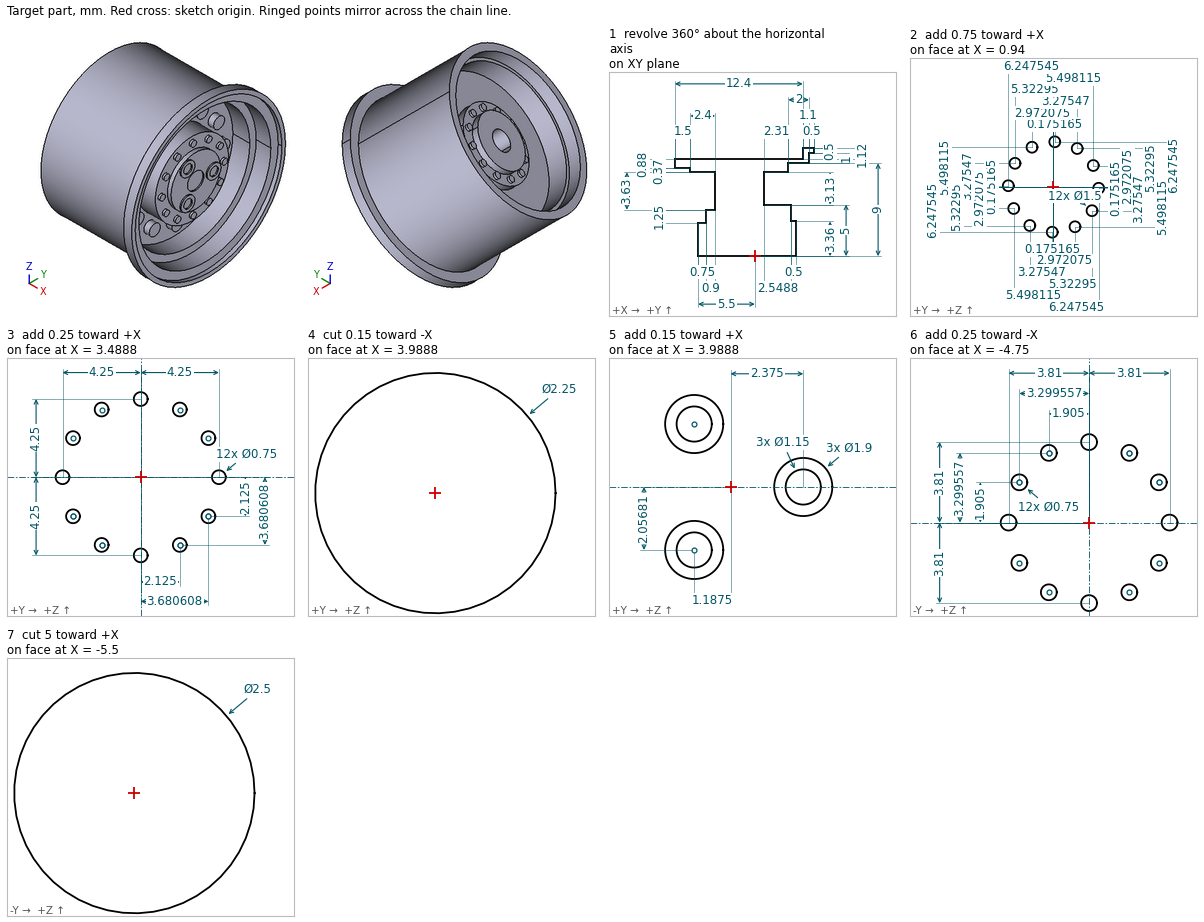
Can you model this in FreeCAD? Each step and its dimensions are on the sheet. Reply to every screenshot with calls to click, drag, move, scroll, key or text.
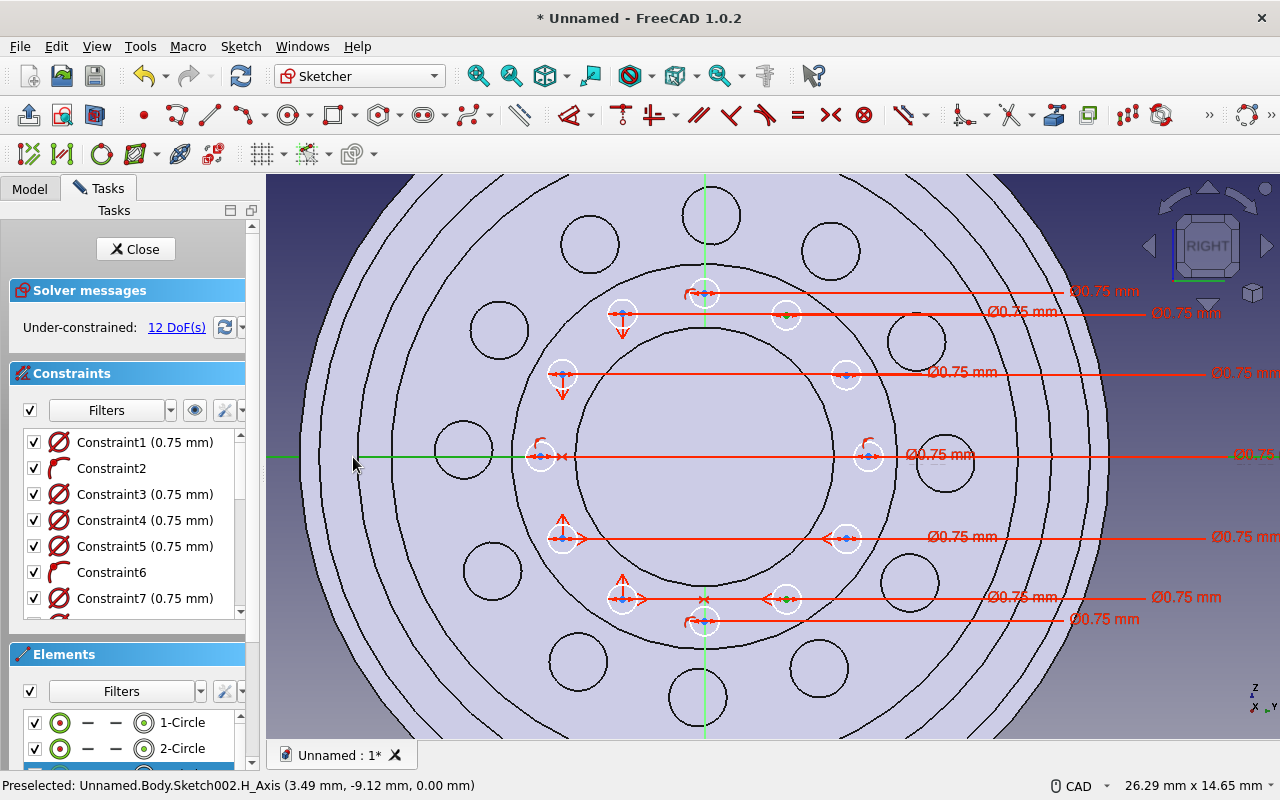
click(831, 116)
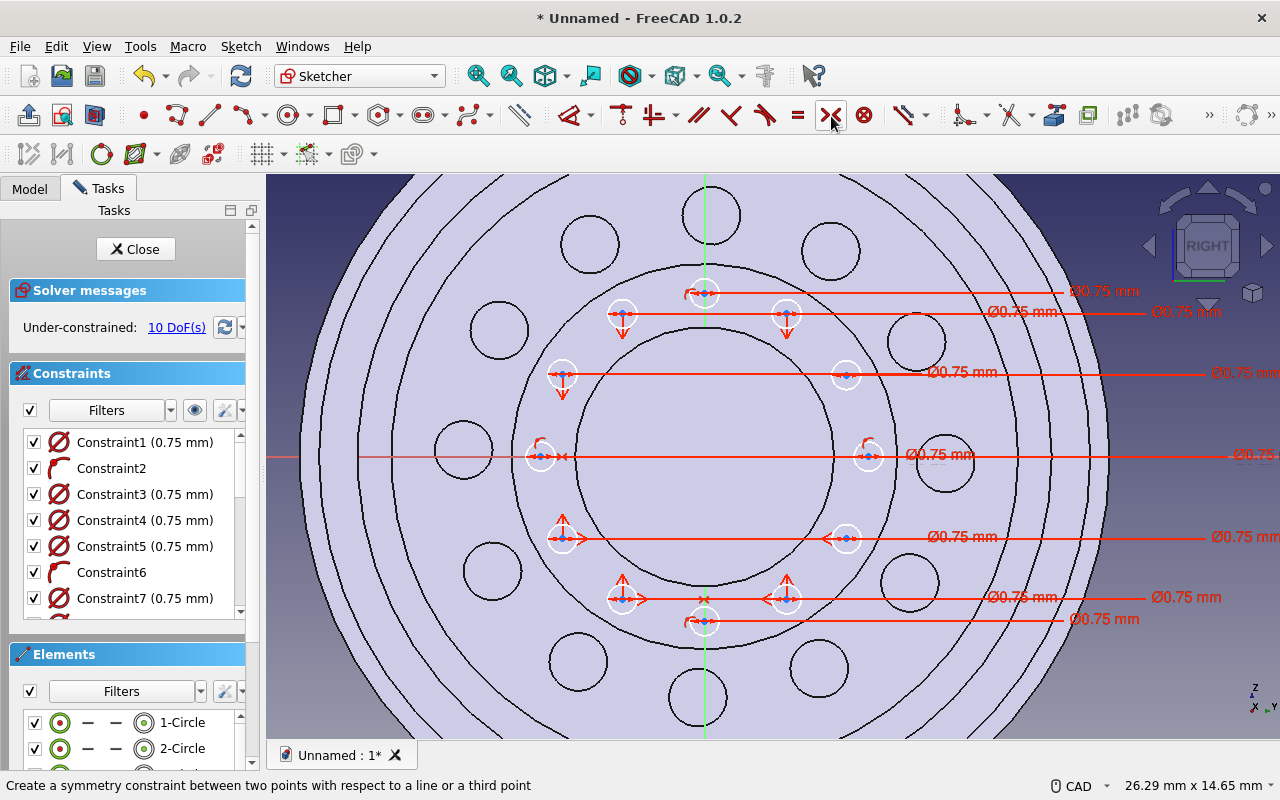
click(847, 539)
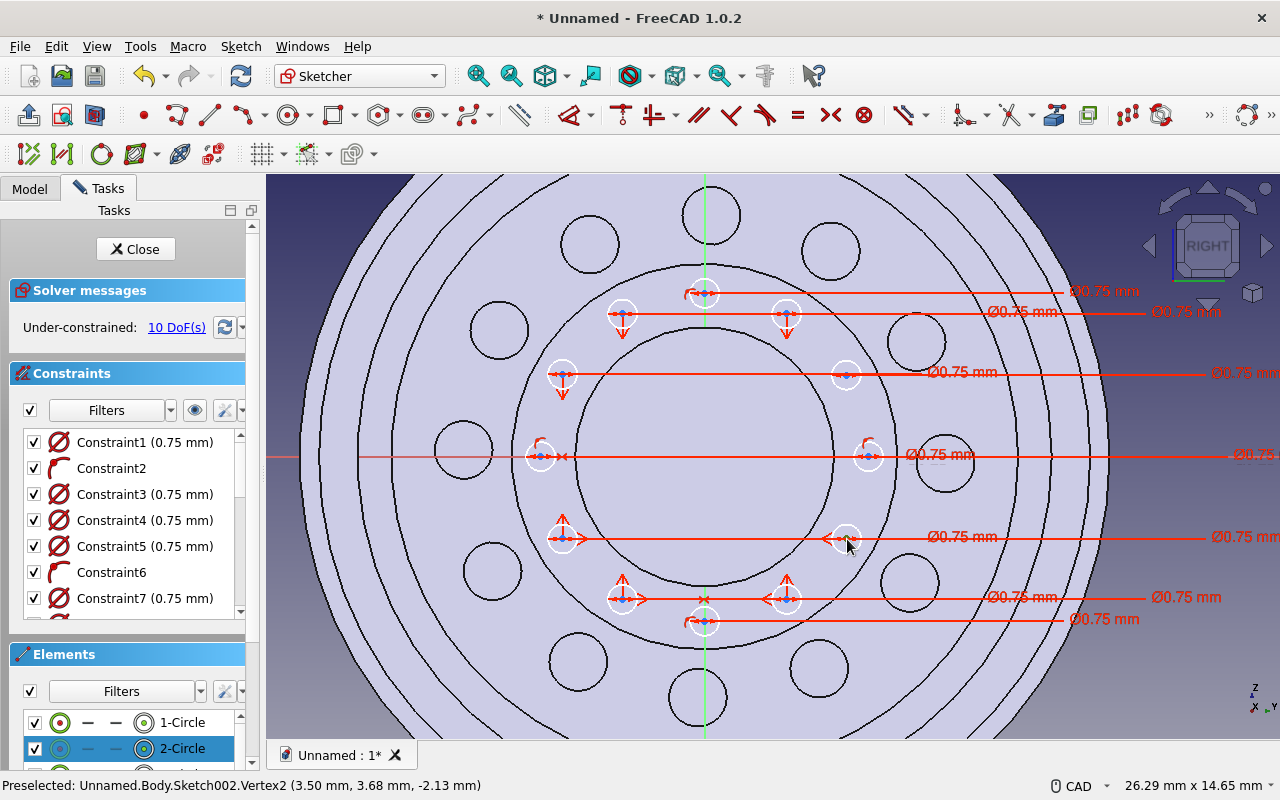
click(846, 375)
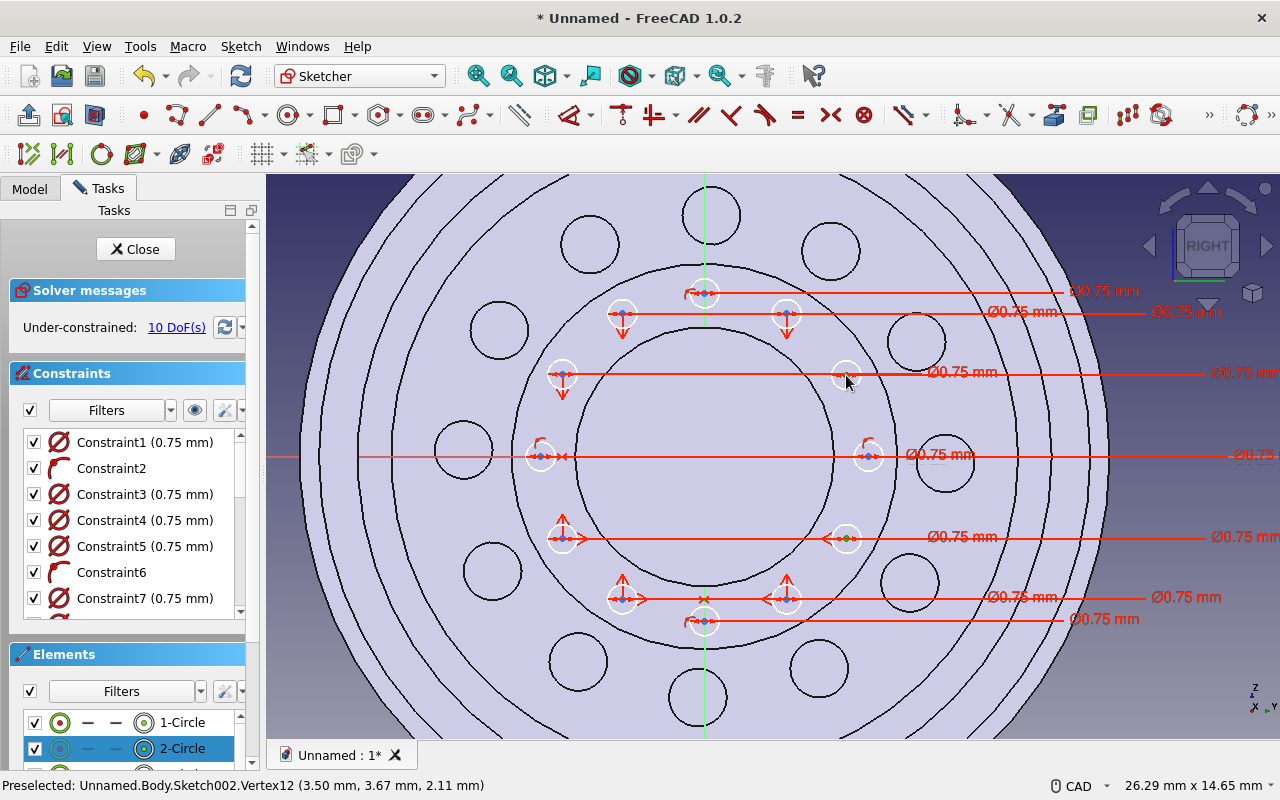
click(353, 457)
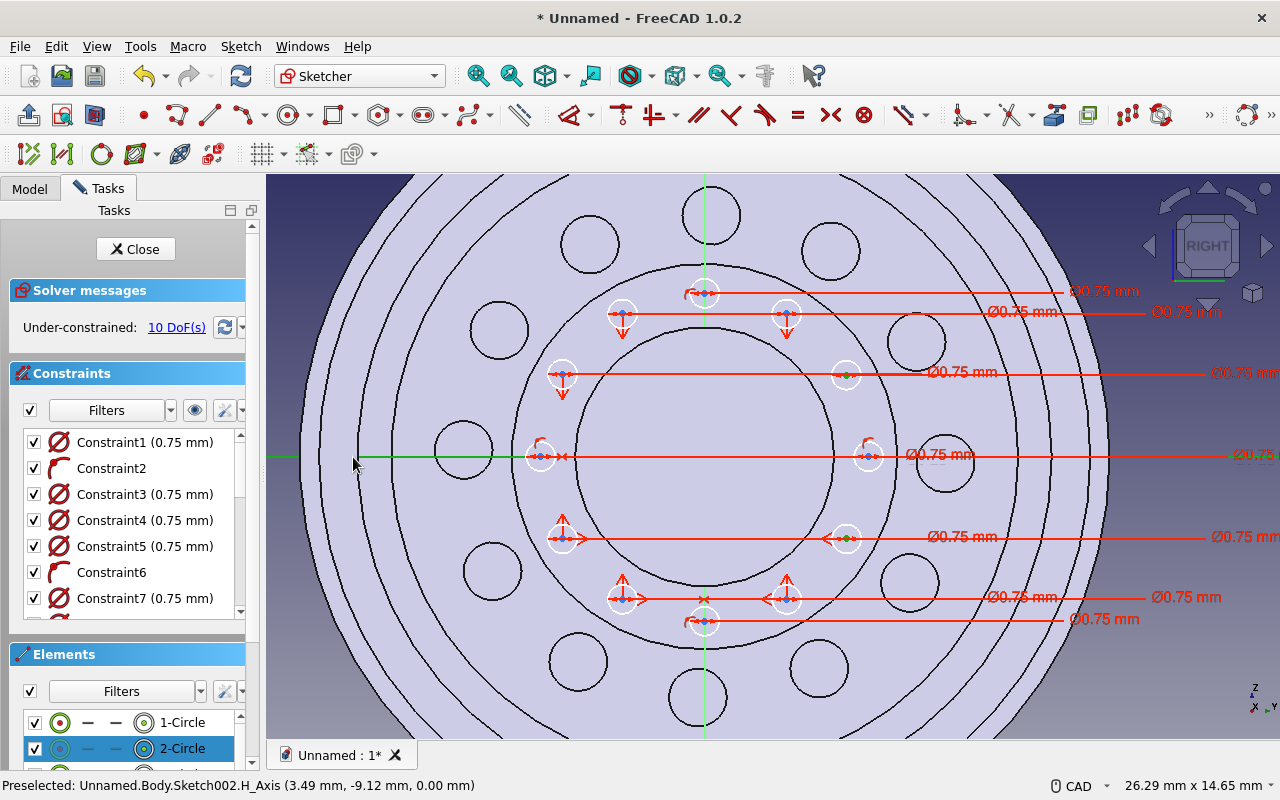
click(831, 116)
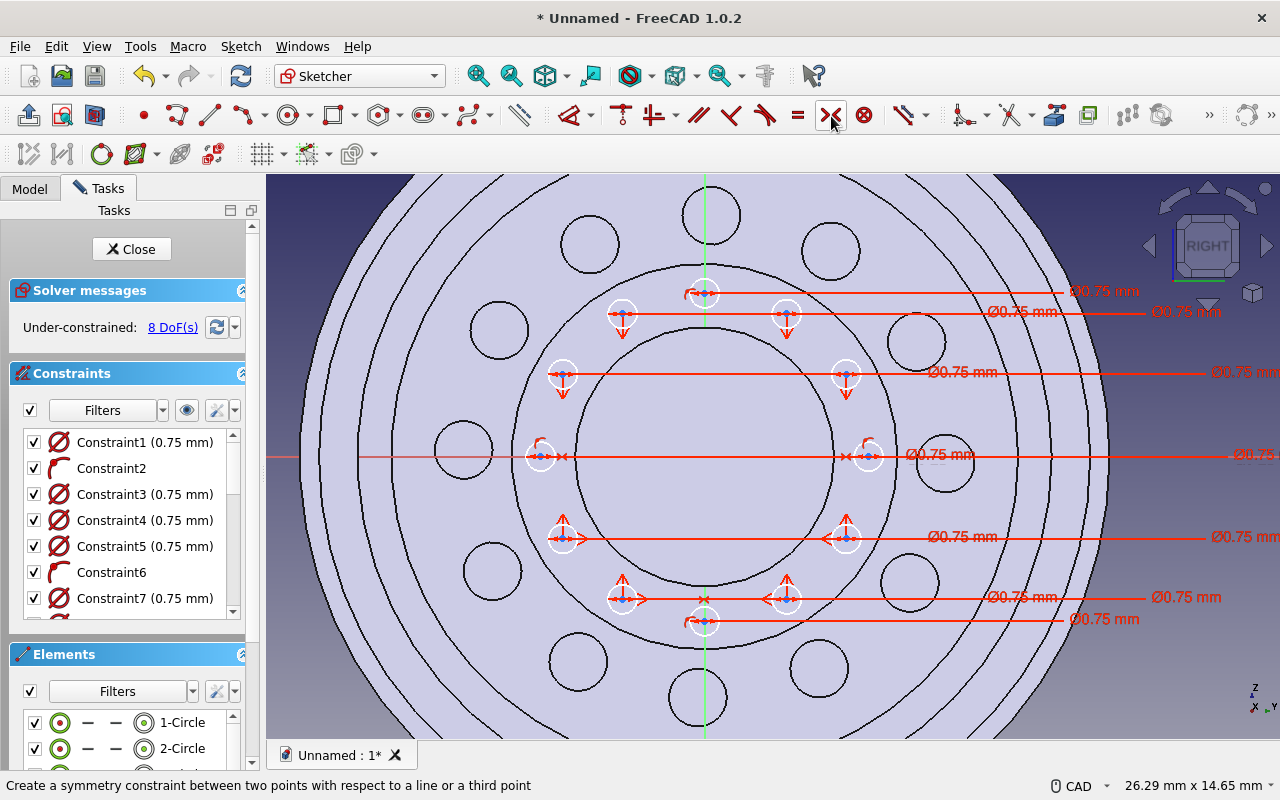
click(568, 116)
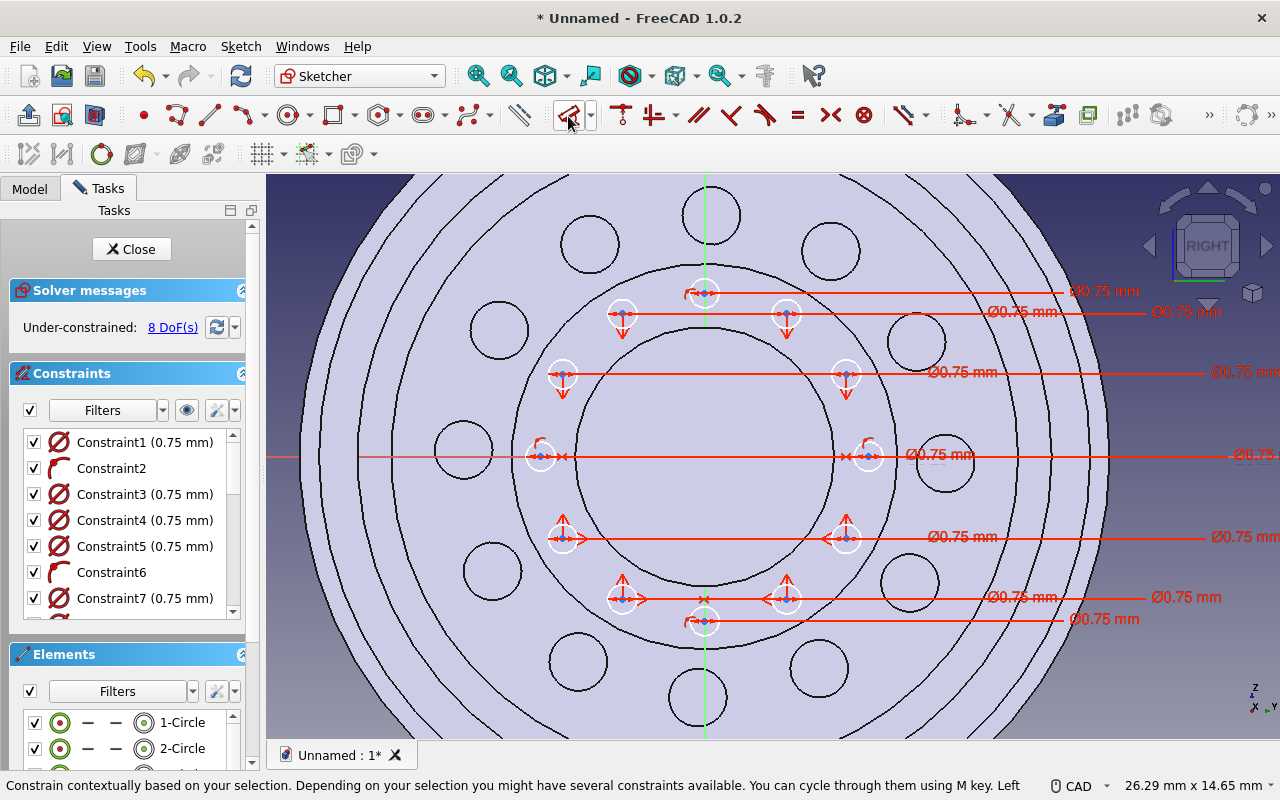
click(869, 457)
click(787, 491)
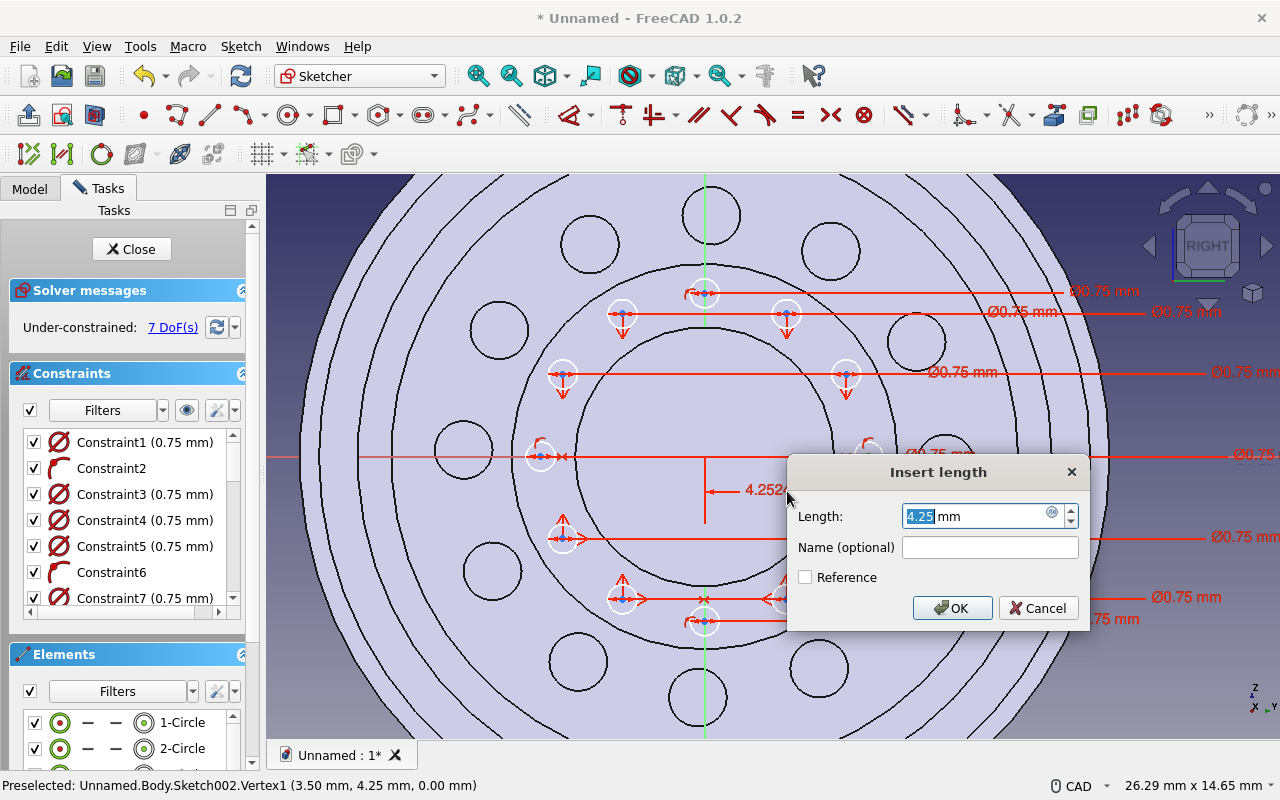
text(4.25)
key(Return)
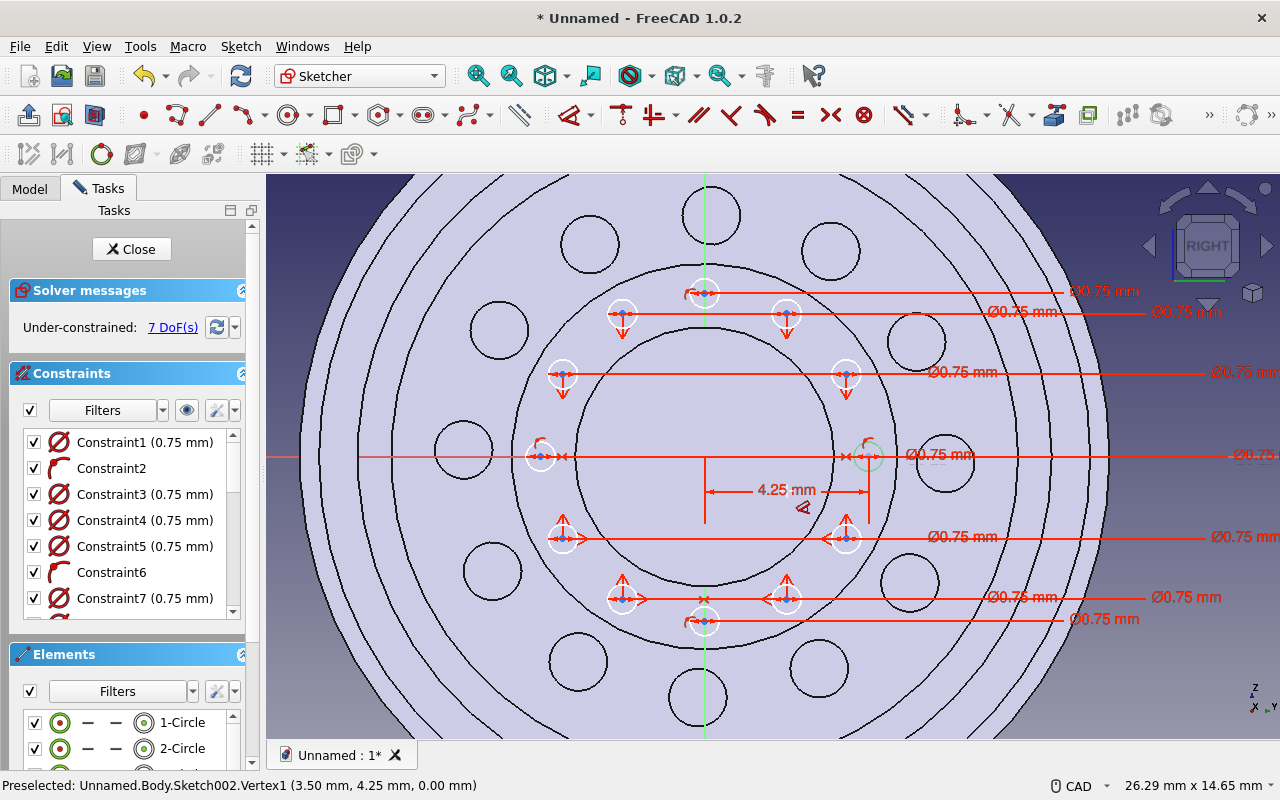
click(705, 621)
click(739, 539)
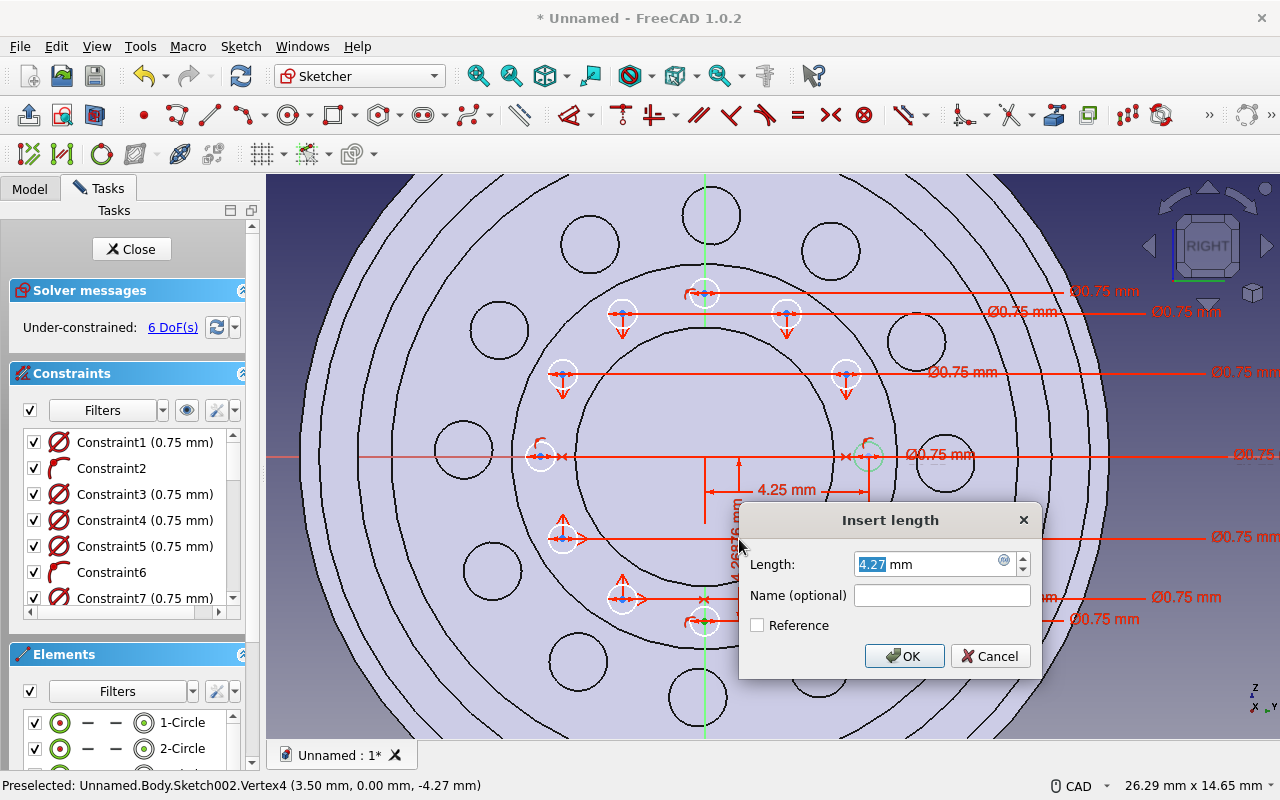
text(4.25)
key(Return)